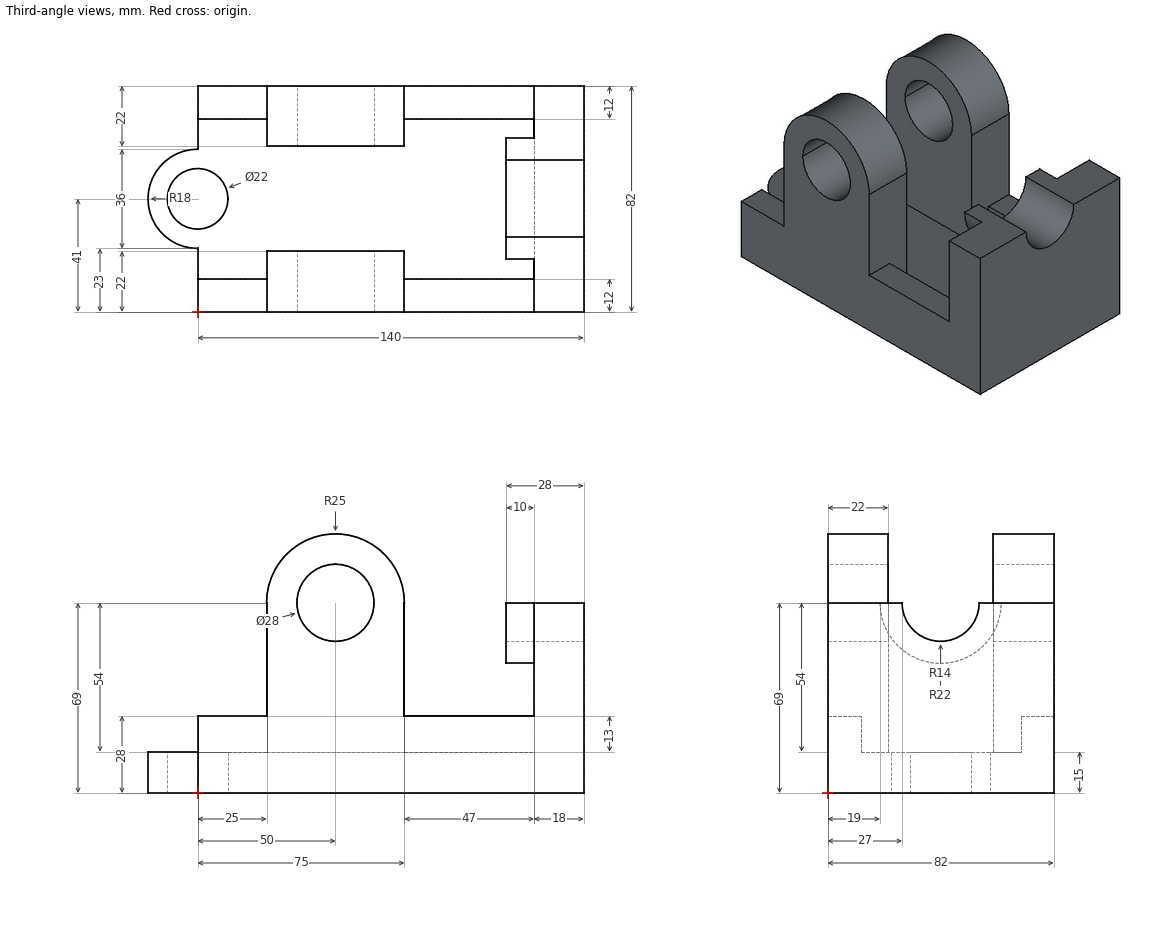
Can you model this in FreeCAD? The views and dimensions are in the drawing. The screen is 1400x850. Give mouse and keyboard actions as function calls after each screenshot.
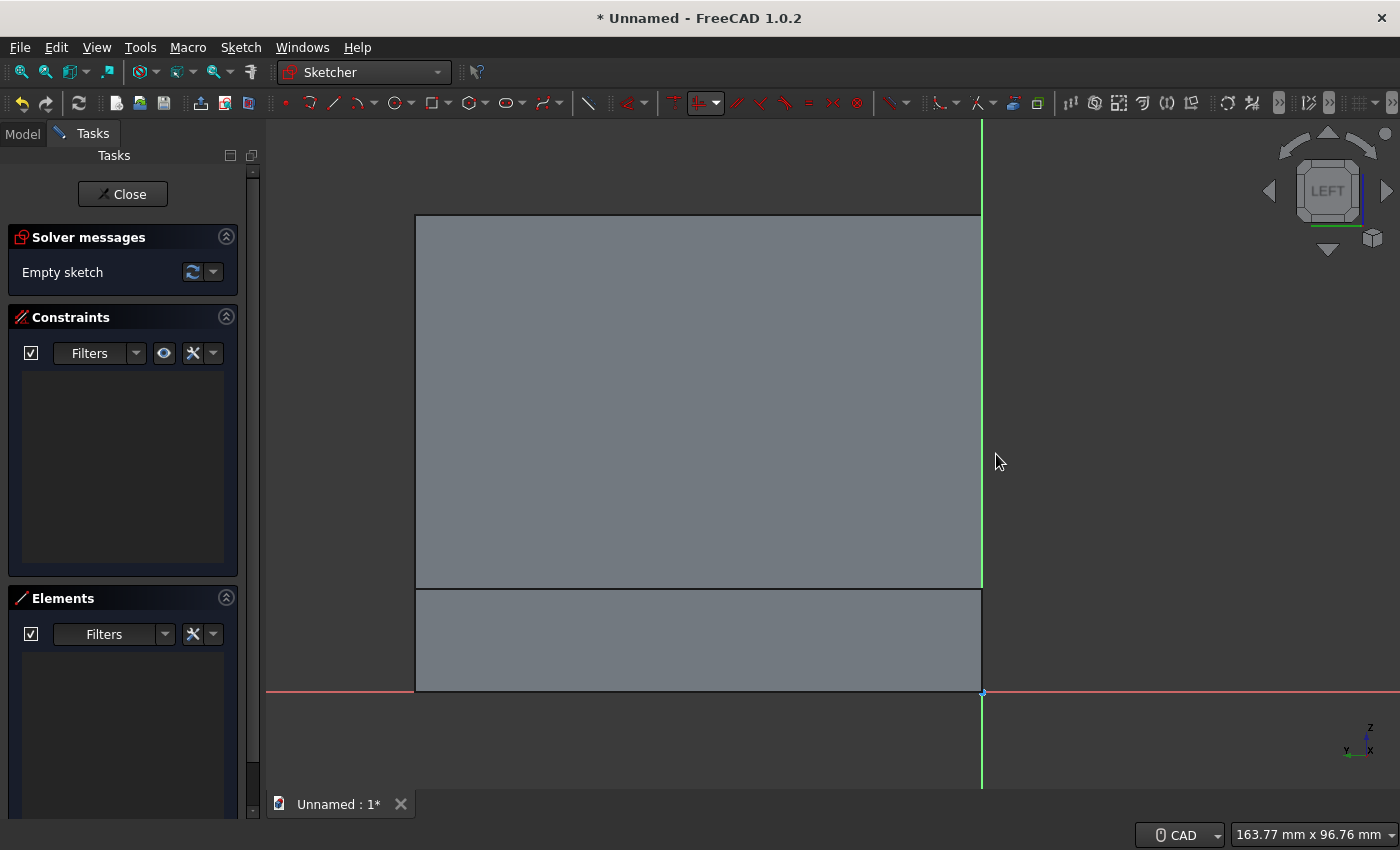
click(334, 104)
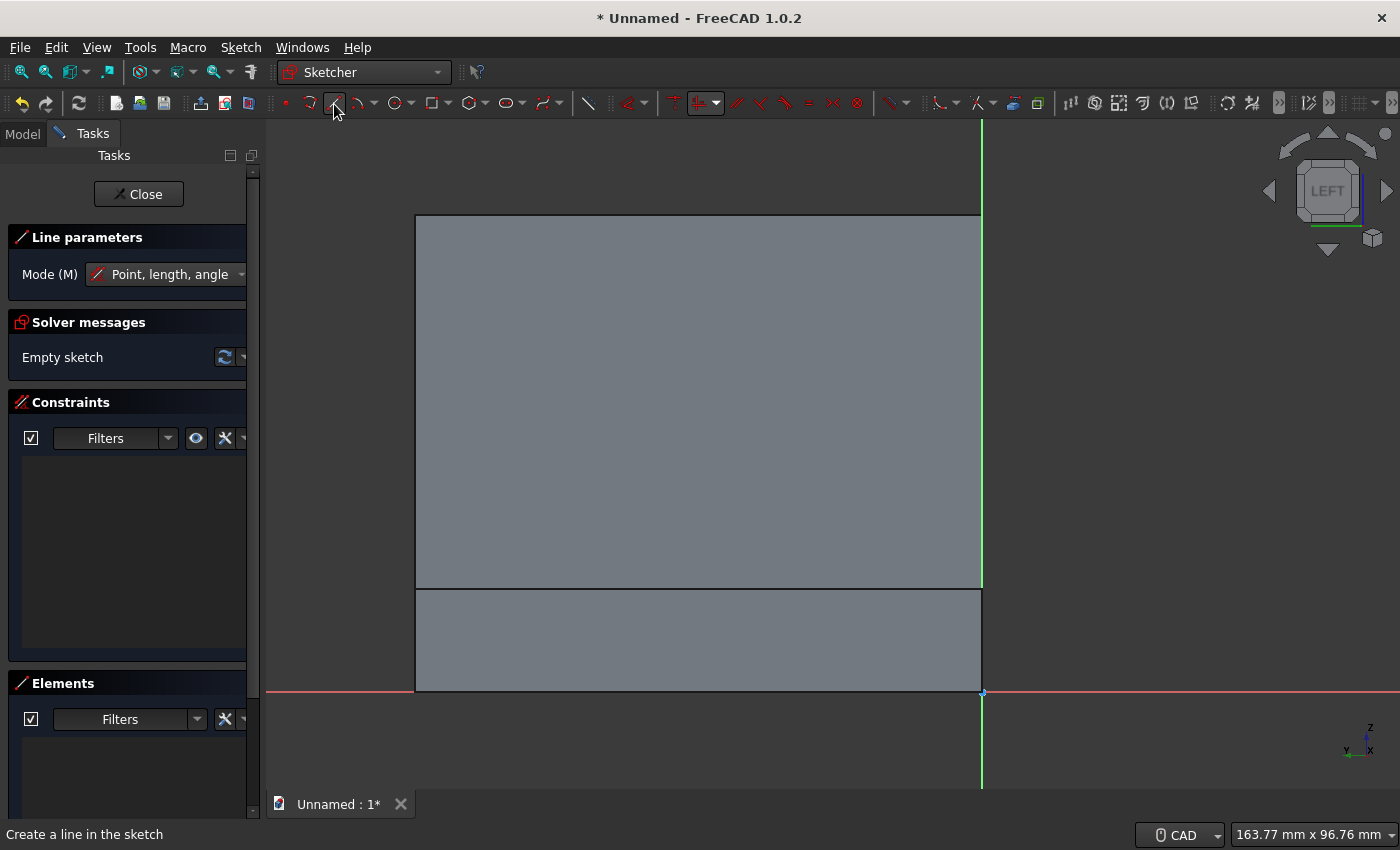
click(851, 215)
click(546, 215)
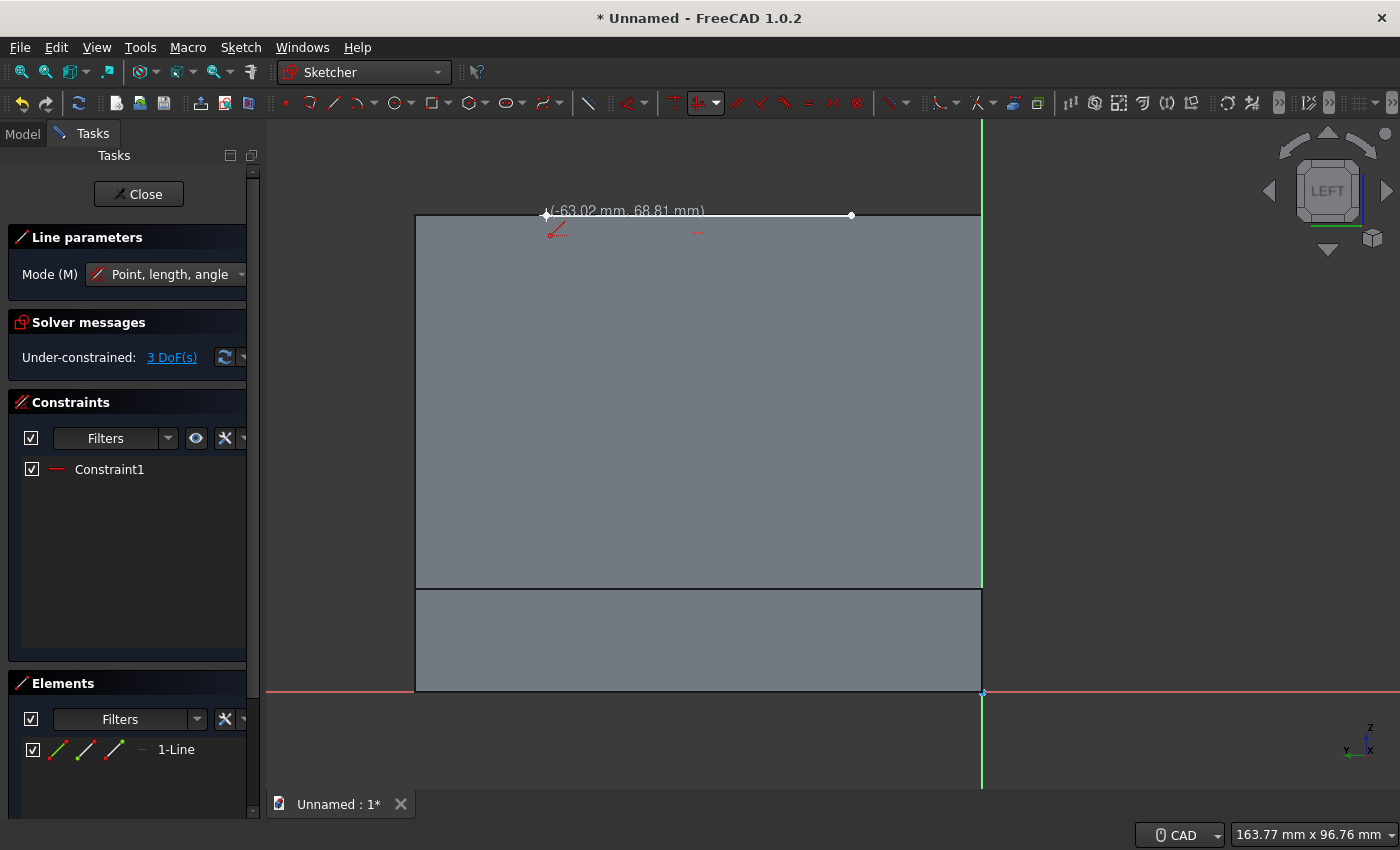
click(376, 104)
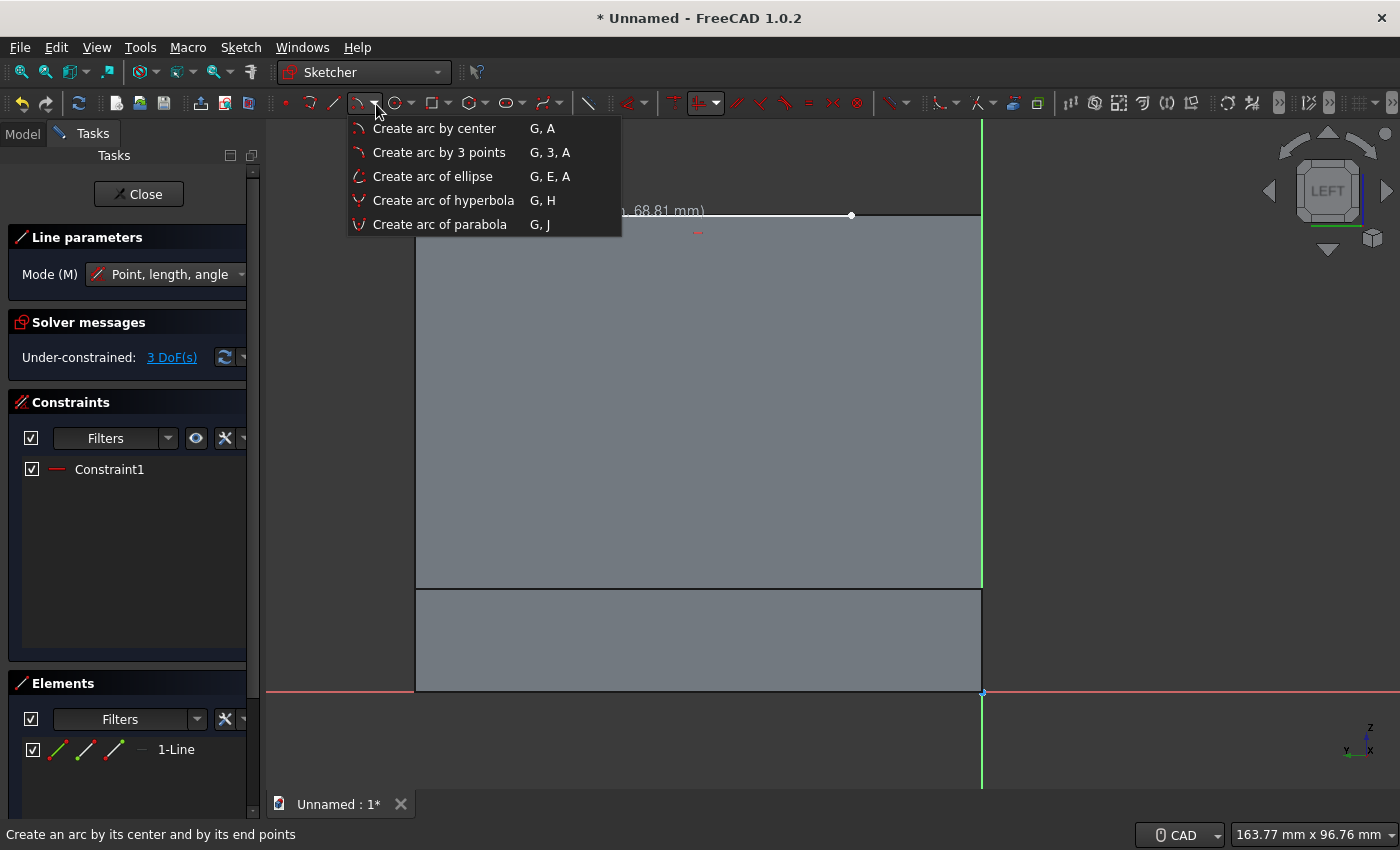
click(484, 152)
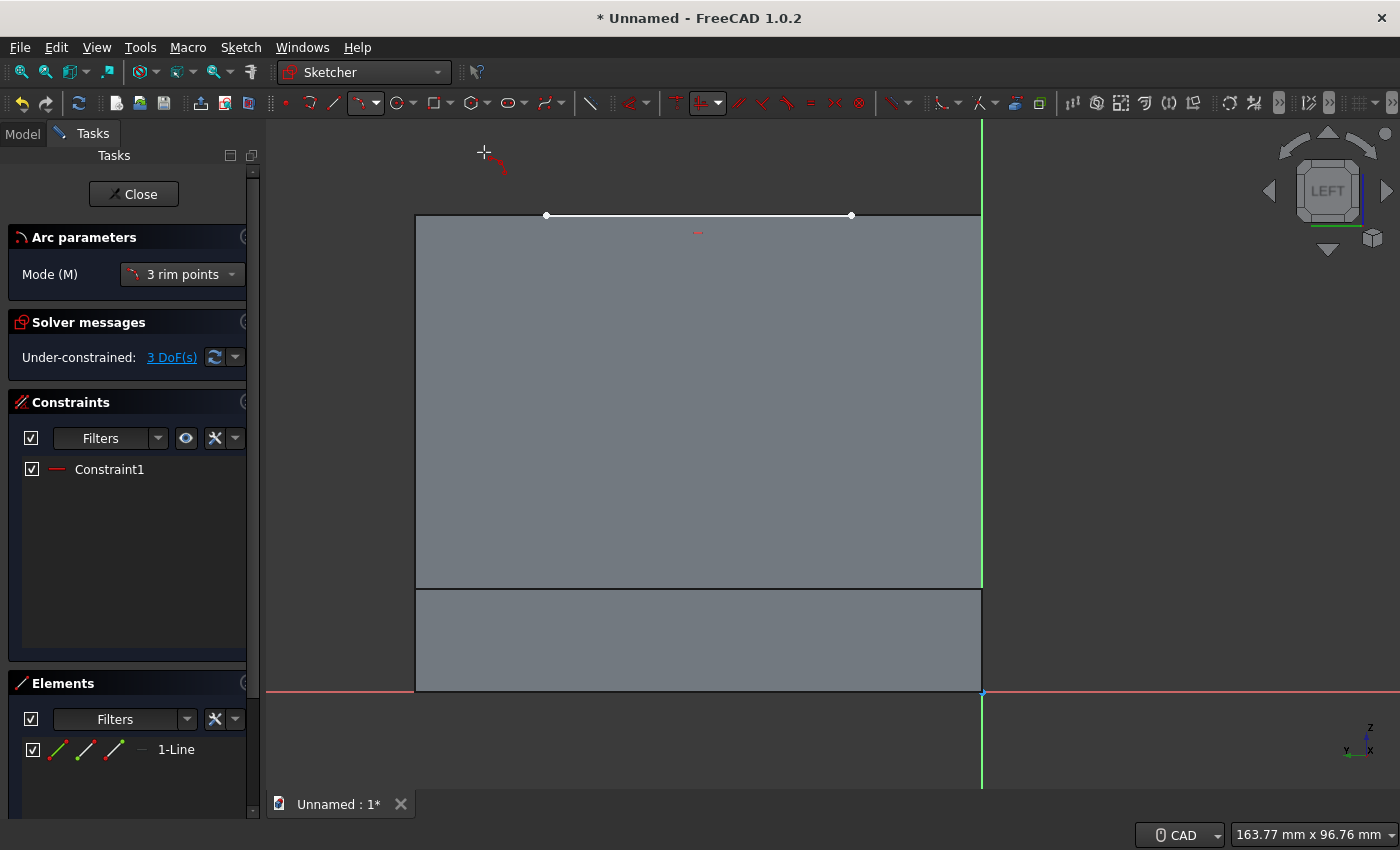
click(546, 216)
click(851, 216)
click(698, 367)
key(Escape)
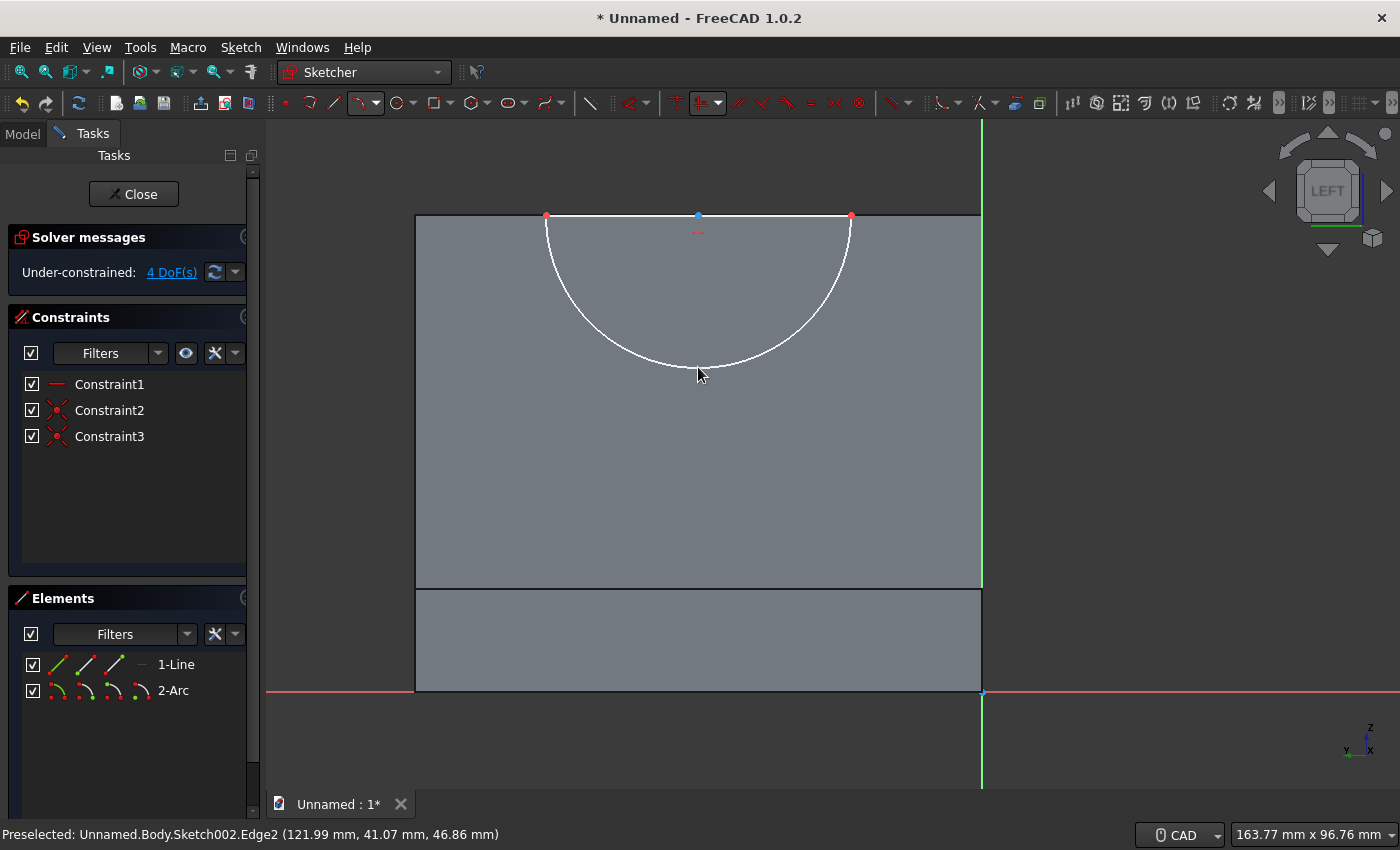
click(630, 104)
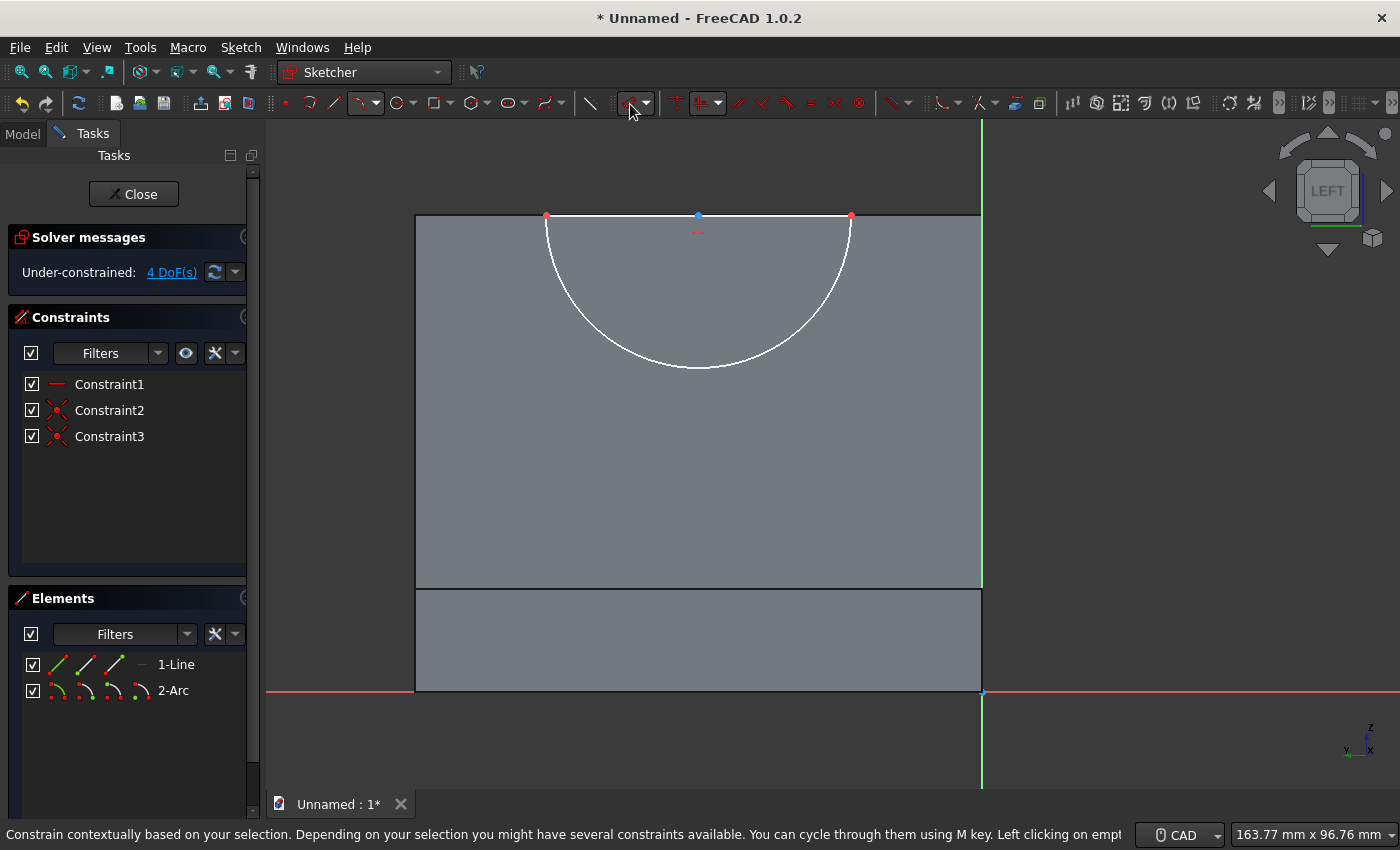
click(609, 339)
click(590, 365)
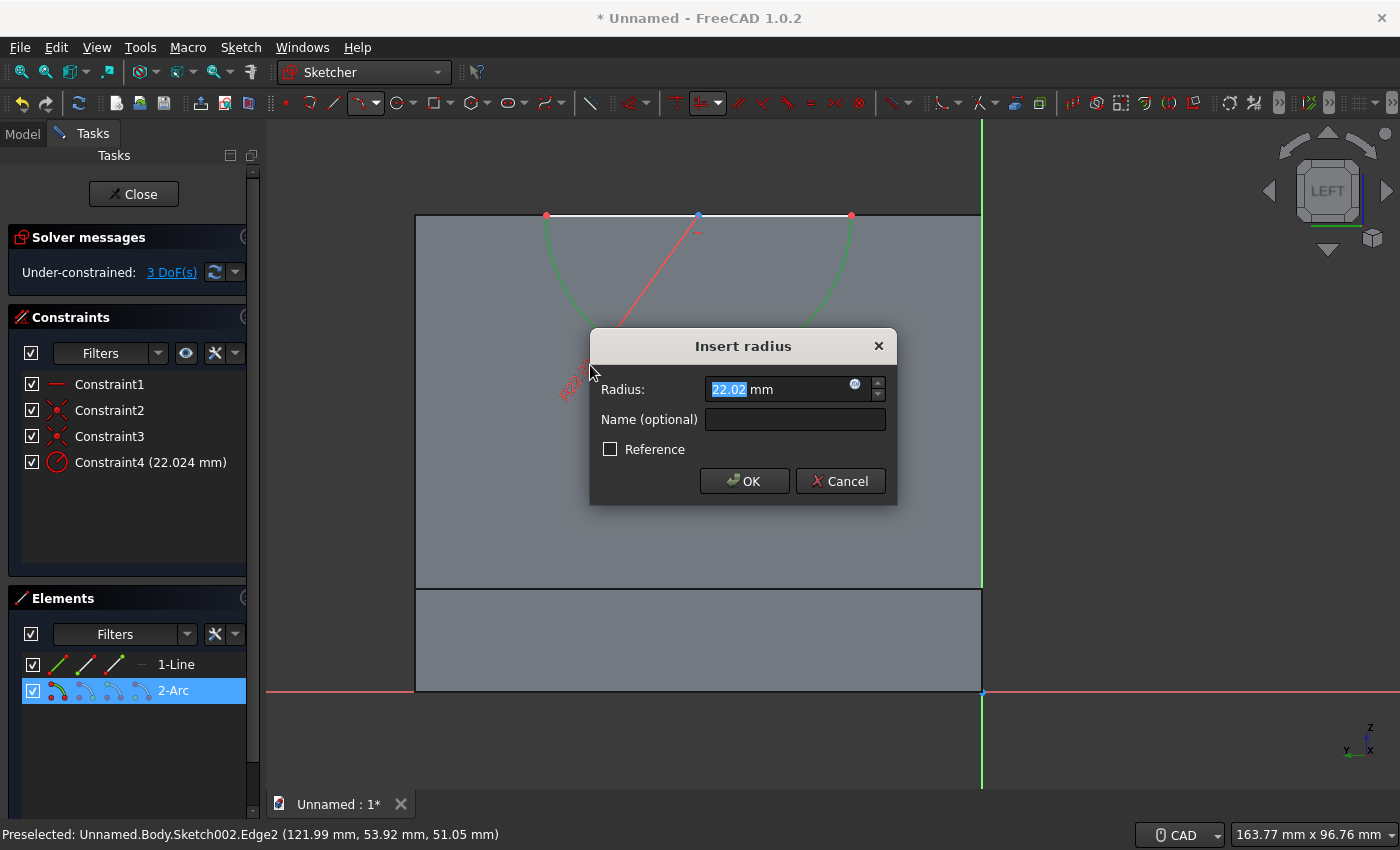
text(22)
key(Return)